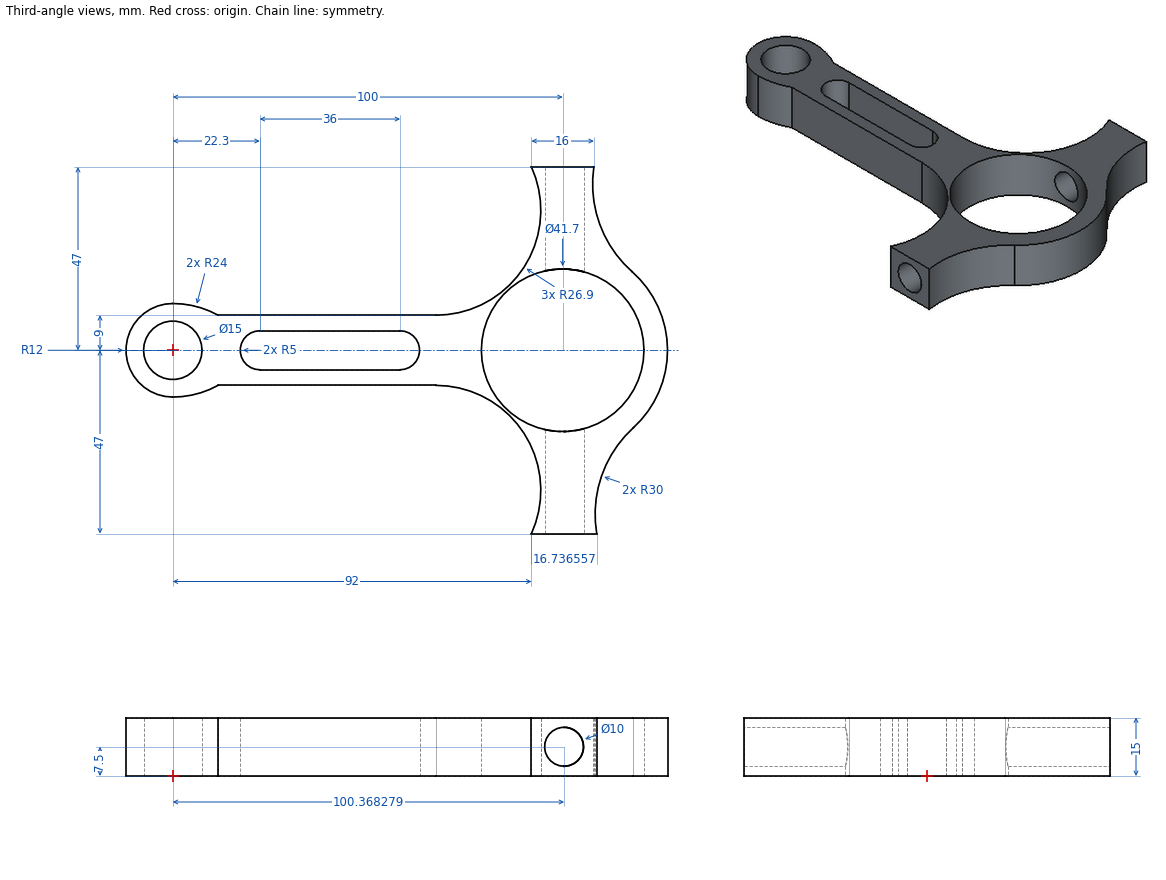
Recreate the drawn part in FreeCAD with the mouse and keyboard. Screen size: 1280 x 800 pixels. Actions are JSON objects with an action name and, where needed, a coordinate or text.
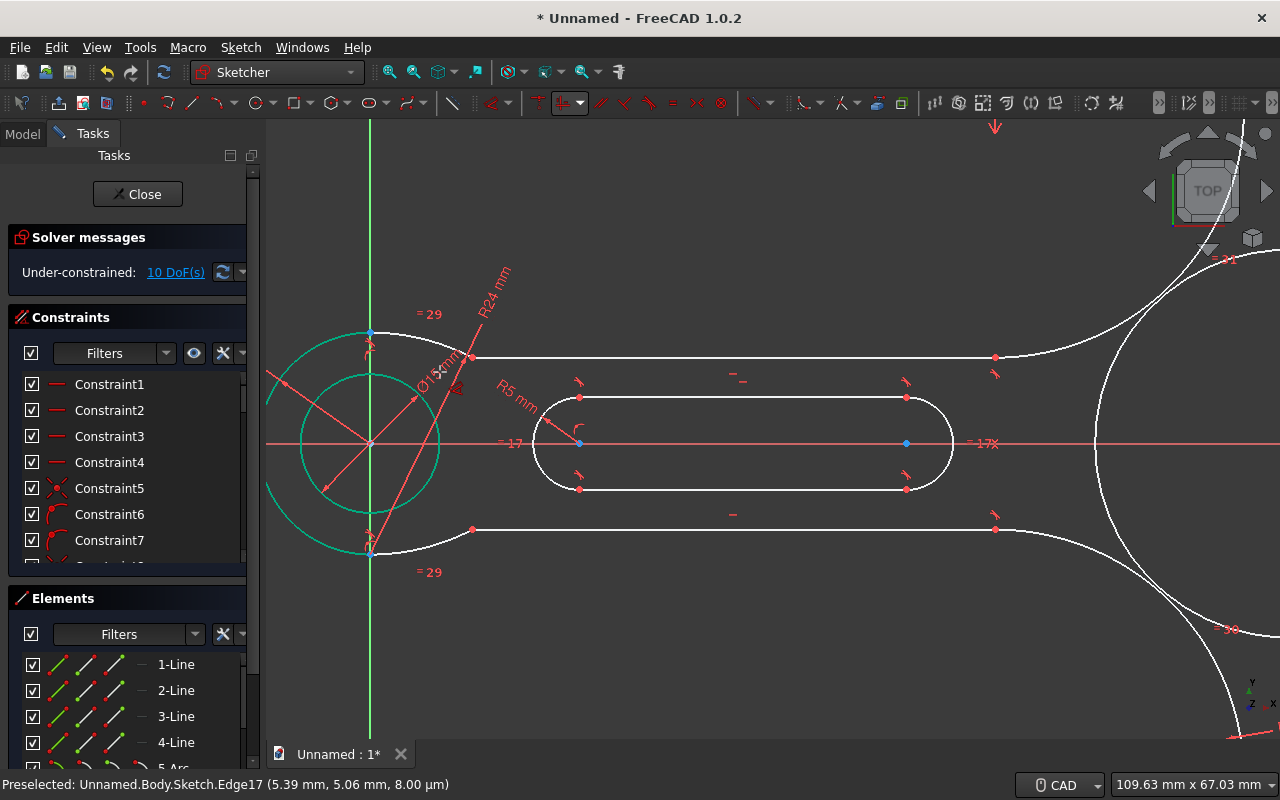
{"action": "scroll", "coordinate": [544, 417], "scroll_direction": "down", "scroll_amount": 4}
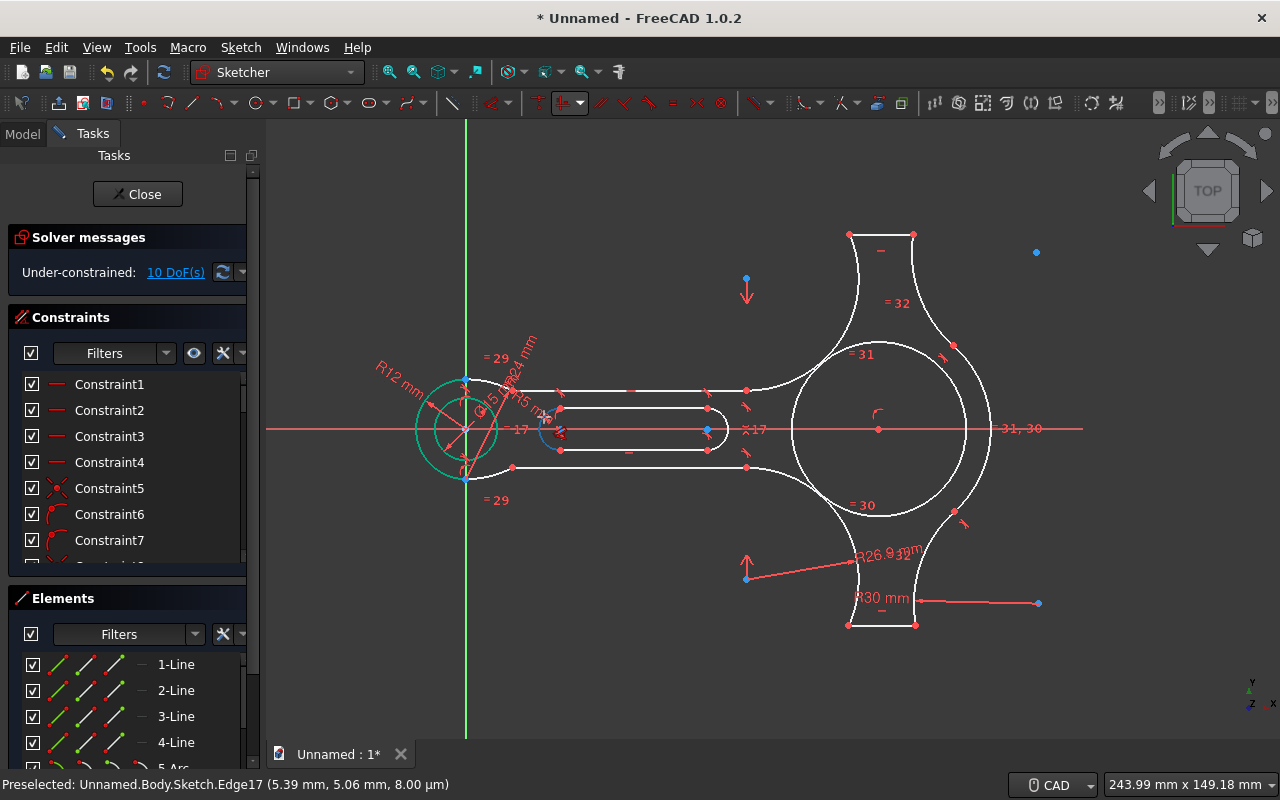
{"action": "left_click", "coordinate": [940, 367]}
{"action": "left_click", "coordinate": [911, 315]}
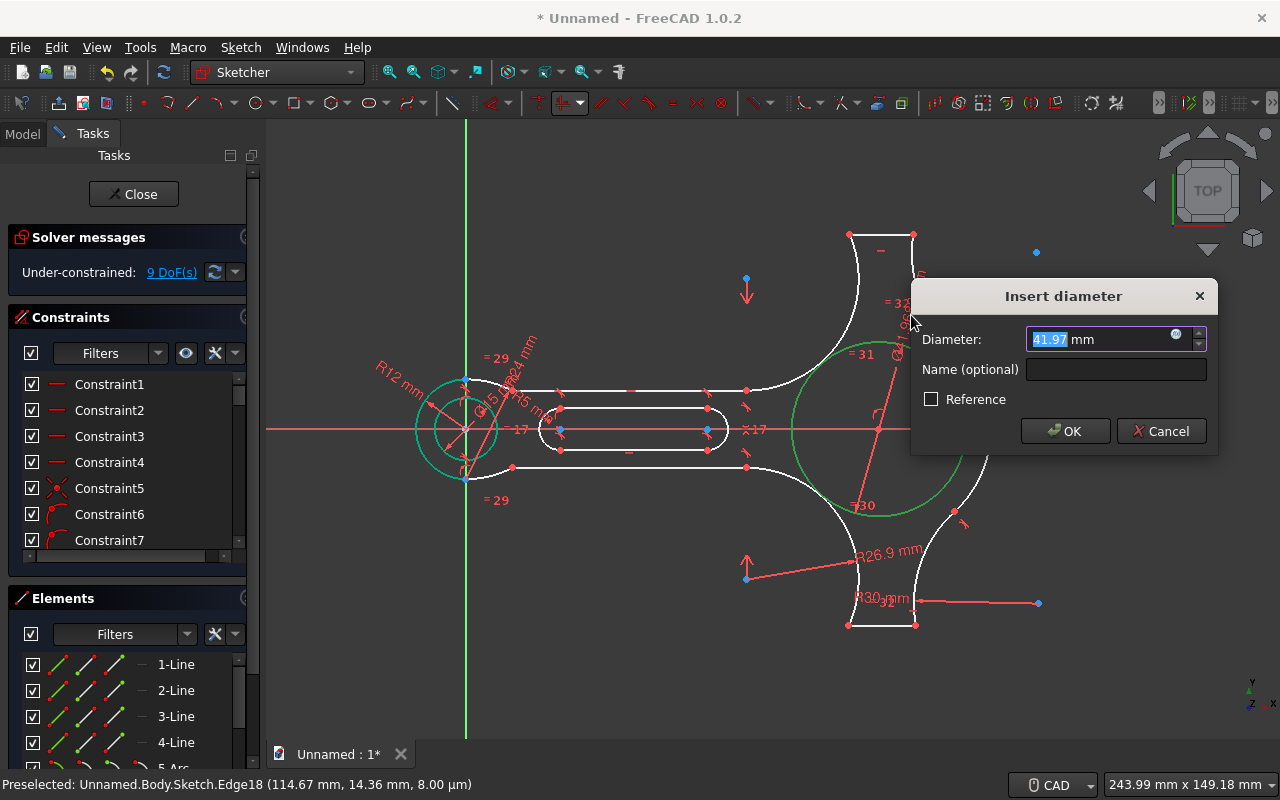
{"action": "type", "text": "41.7"}
{"action": "key", "text": "Return"}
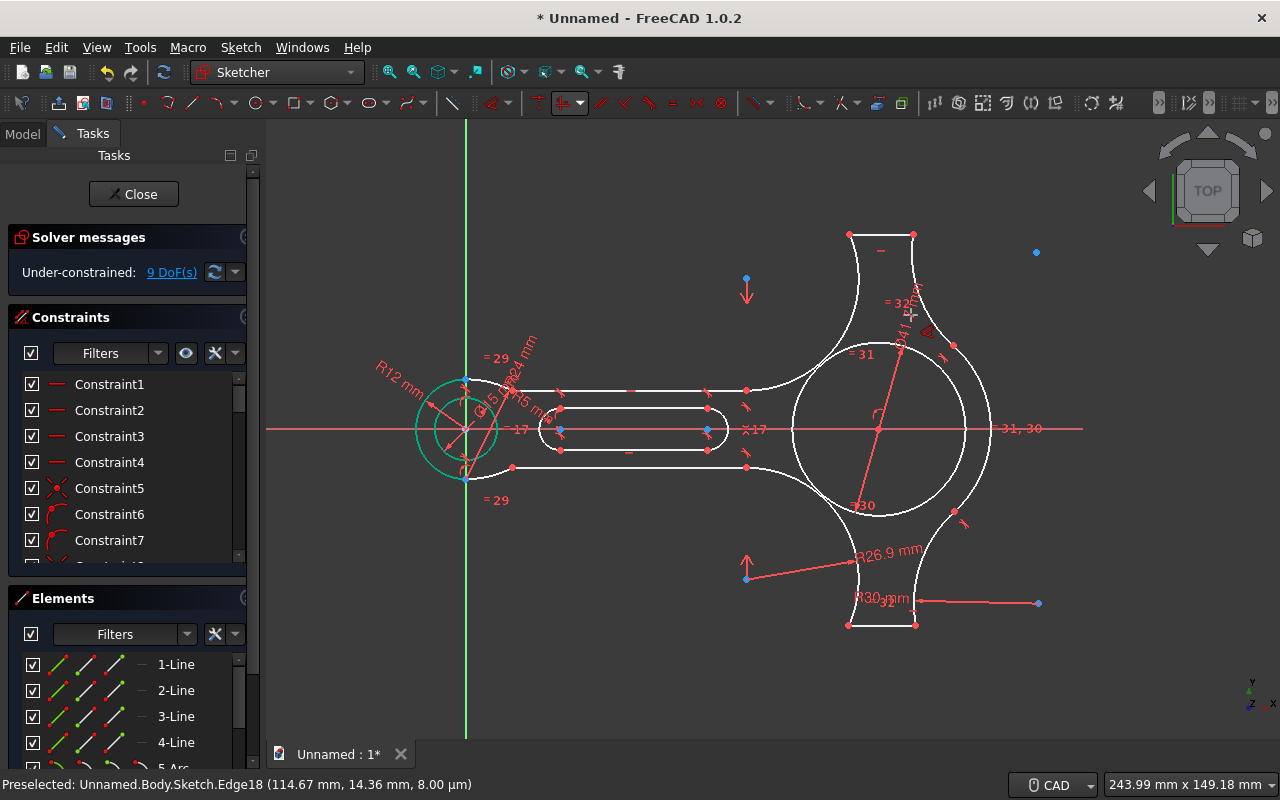
{"action": "left_click", "coordinate": [894, 235]}
{"action": "left_click", "coordinate": [881, 201]}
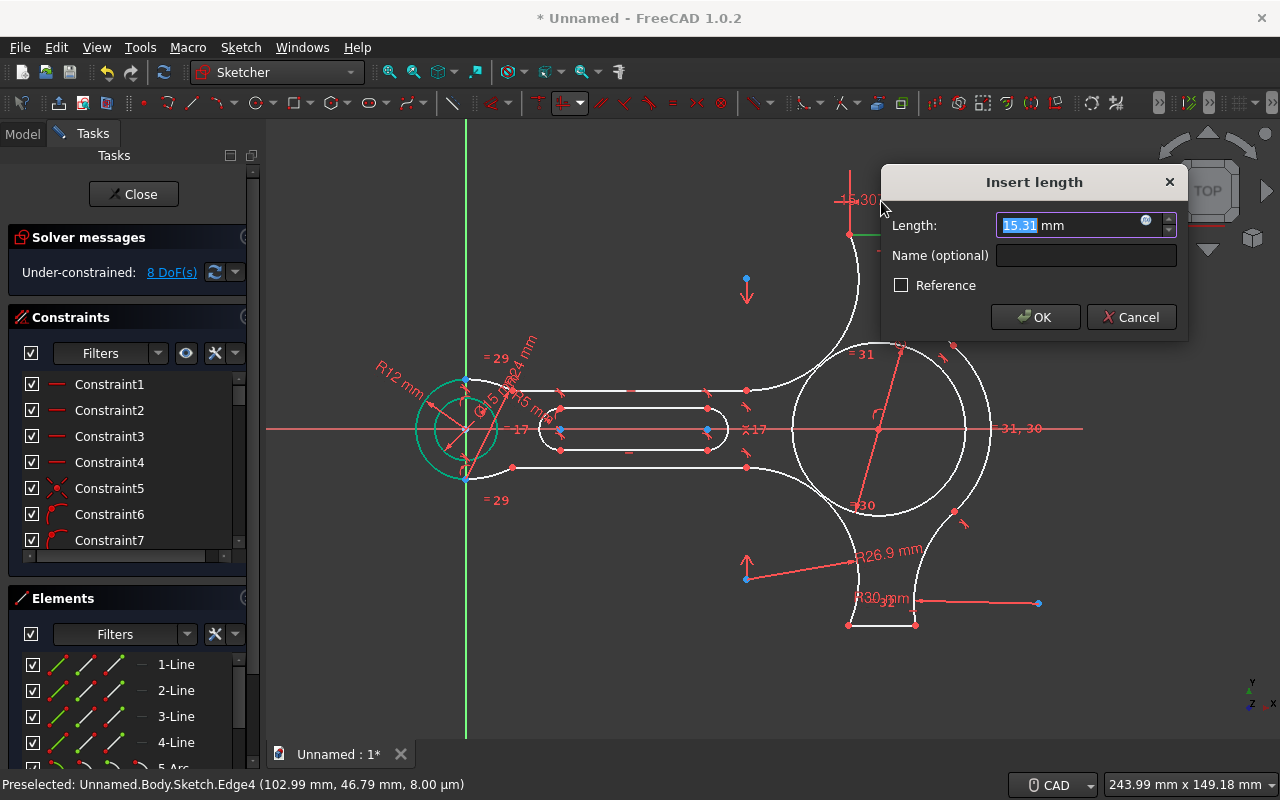
{"action": "type", "text": "16"}
{"action": "key", "text": "Return"}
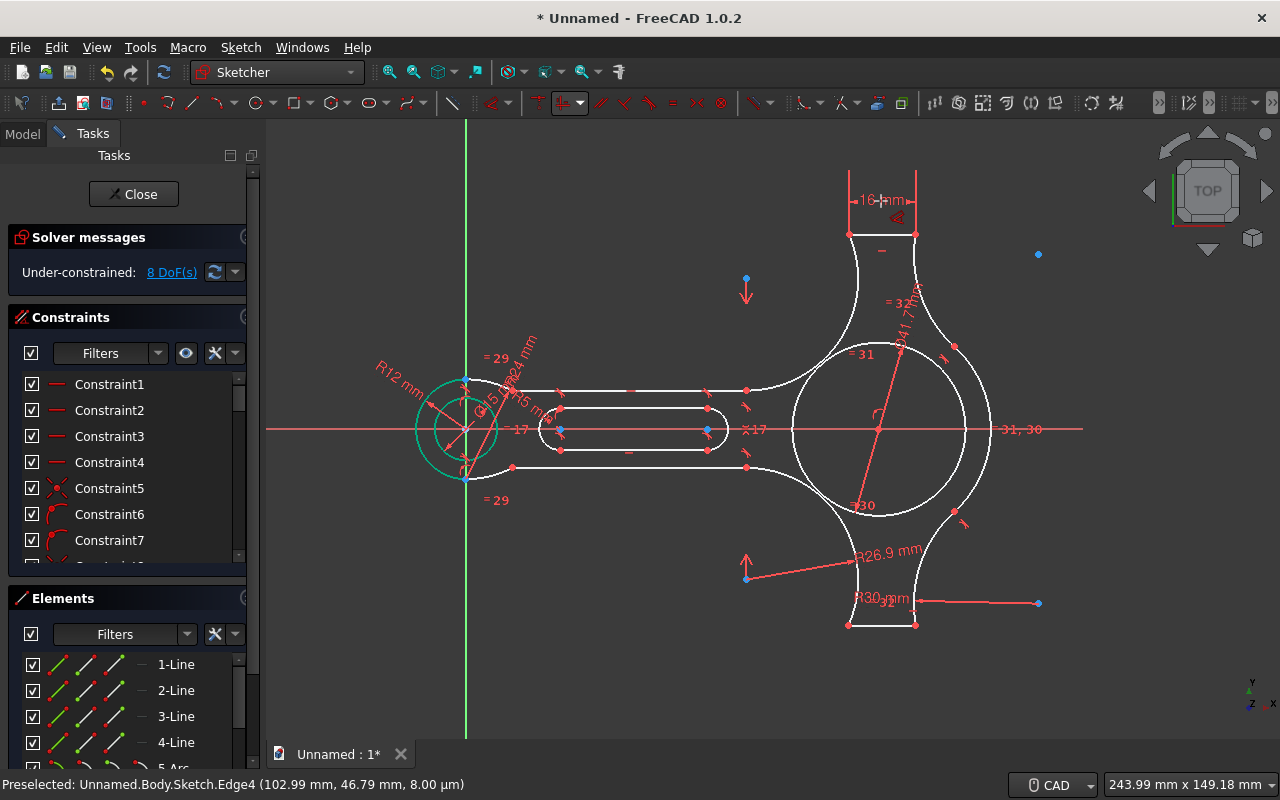
{"action": "left_click", "coordinate": [604, 408]}
{"action": "left_click", "coordinate": [634, 374]}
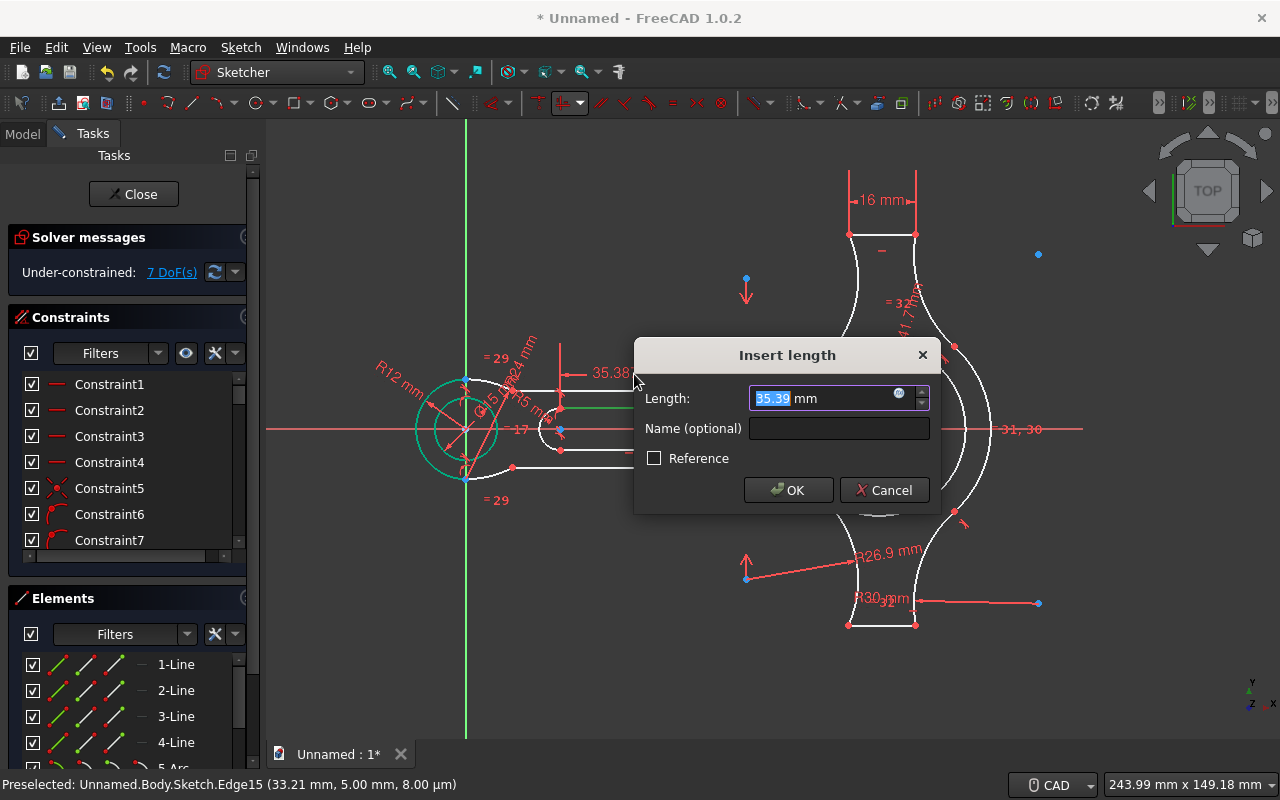
{"action": "type", "text": "36"}
{"action": "key", "text": "Return"}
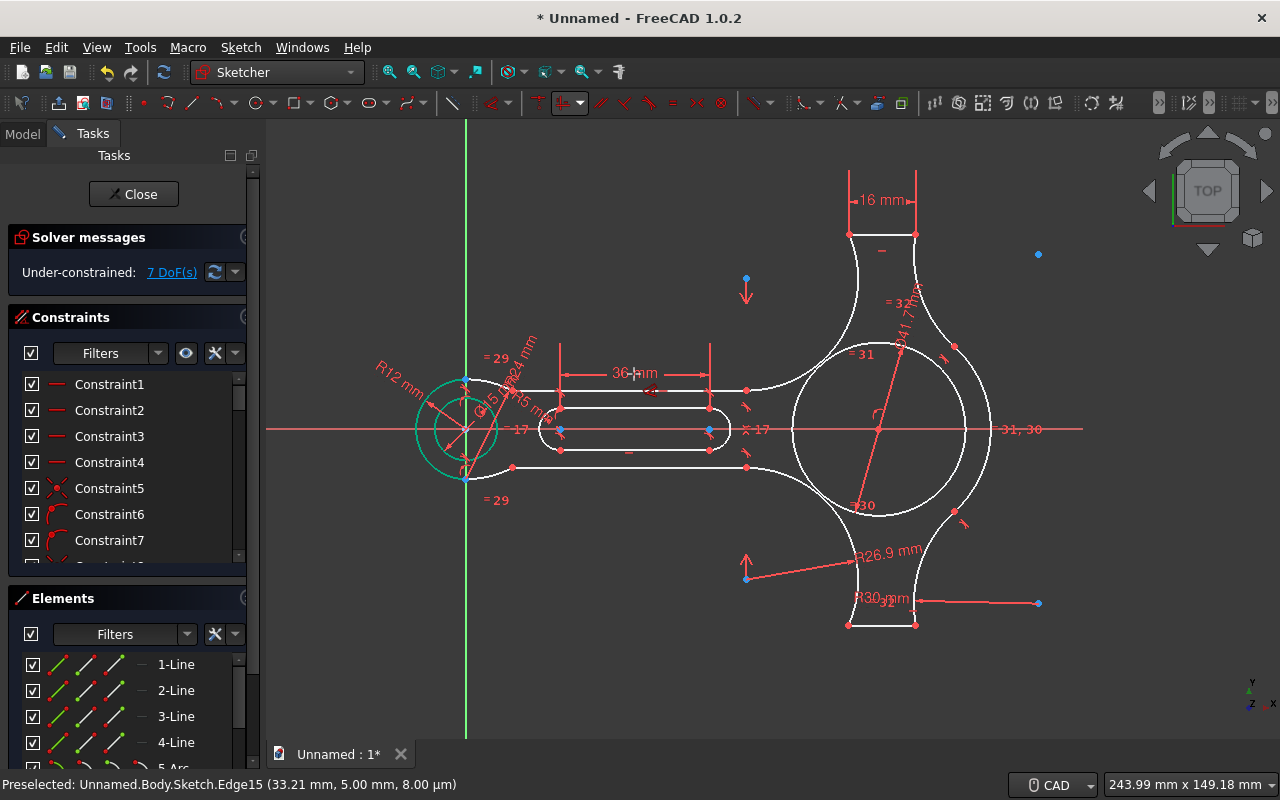
{"action": "left_click", "coordinate": [746, 391]}
{"action": "left_click", "coordinate": [780, 410]}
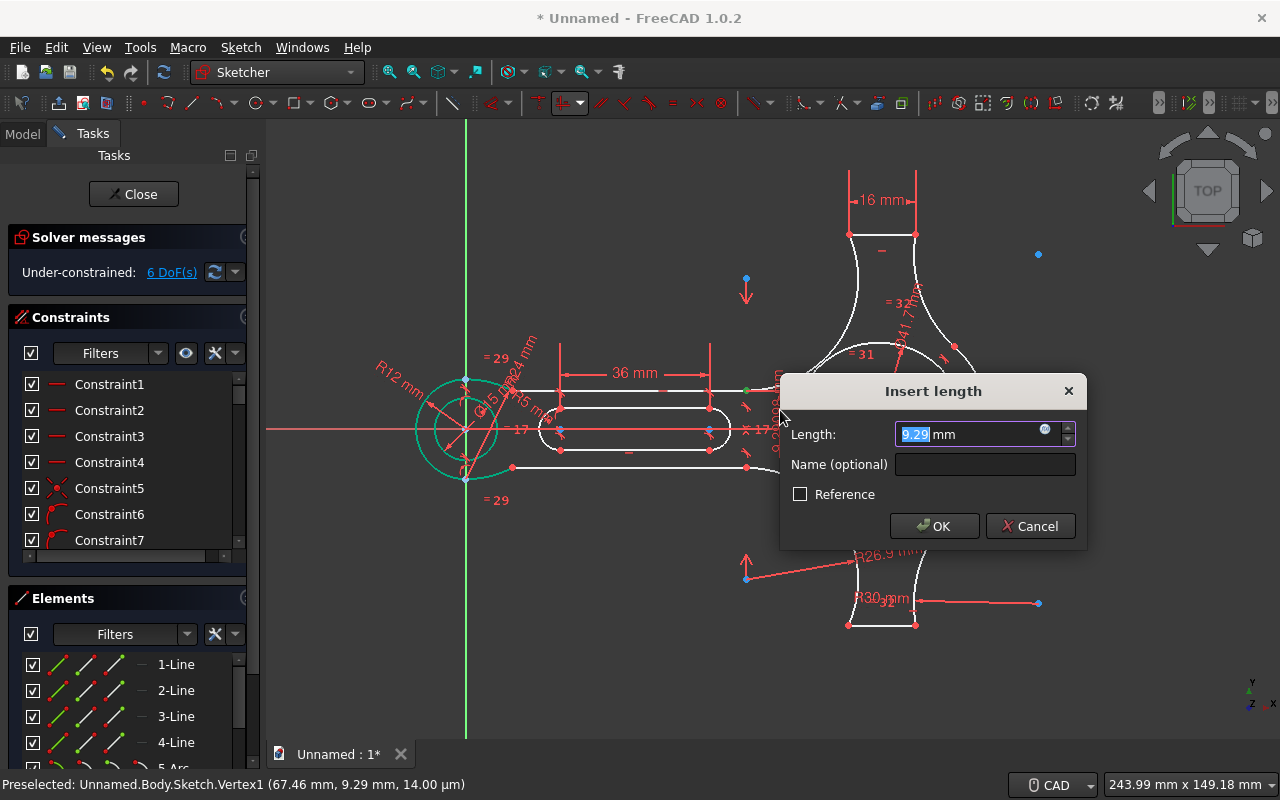
{"action": "type", "text": "9"}
{"action": "key", "text": "Return"}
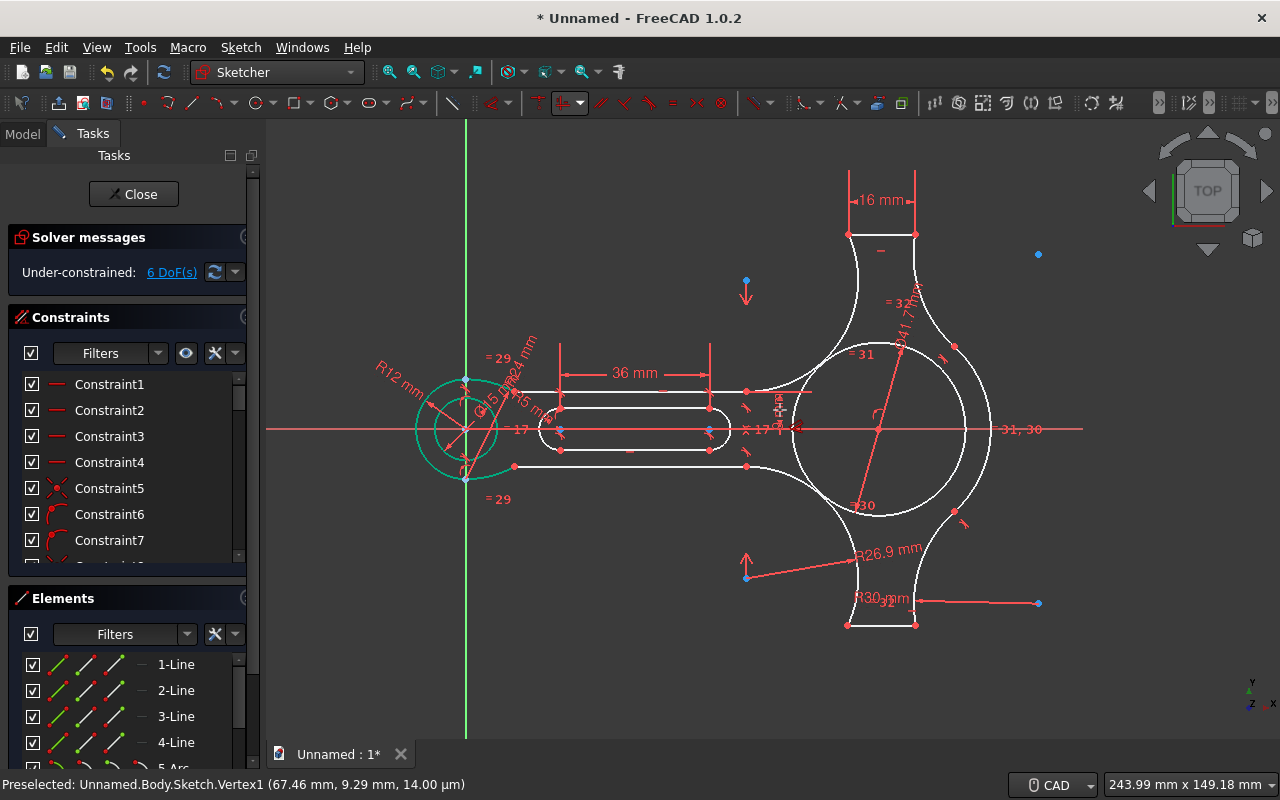
{"action": "left_click", "coordinate": [848, 626]}
{"action": "left_click", "coordinate": [657, 660]}